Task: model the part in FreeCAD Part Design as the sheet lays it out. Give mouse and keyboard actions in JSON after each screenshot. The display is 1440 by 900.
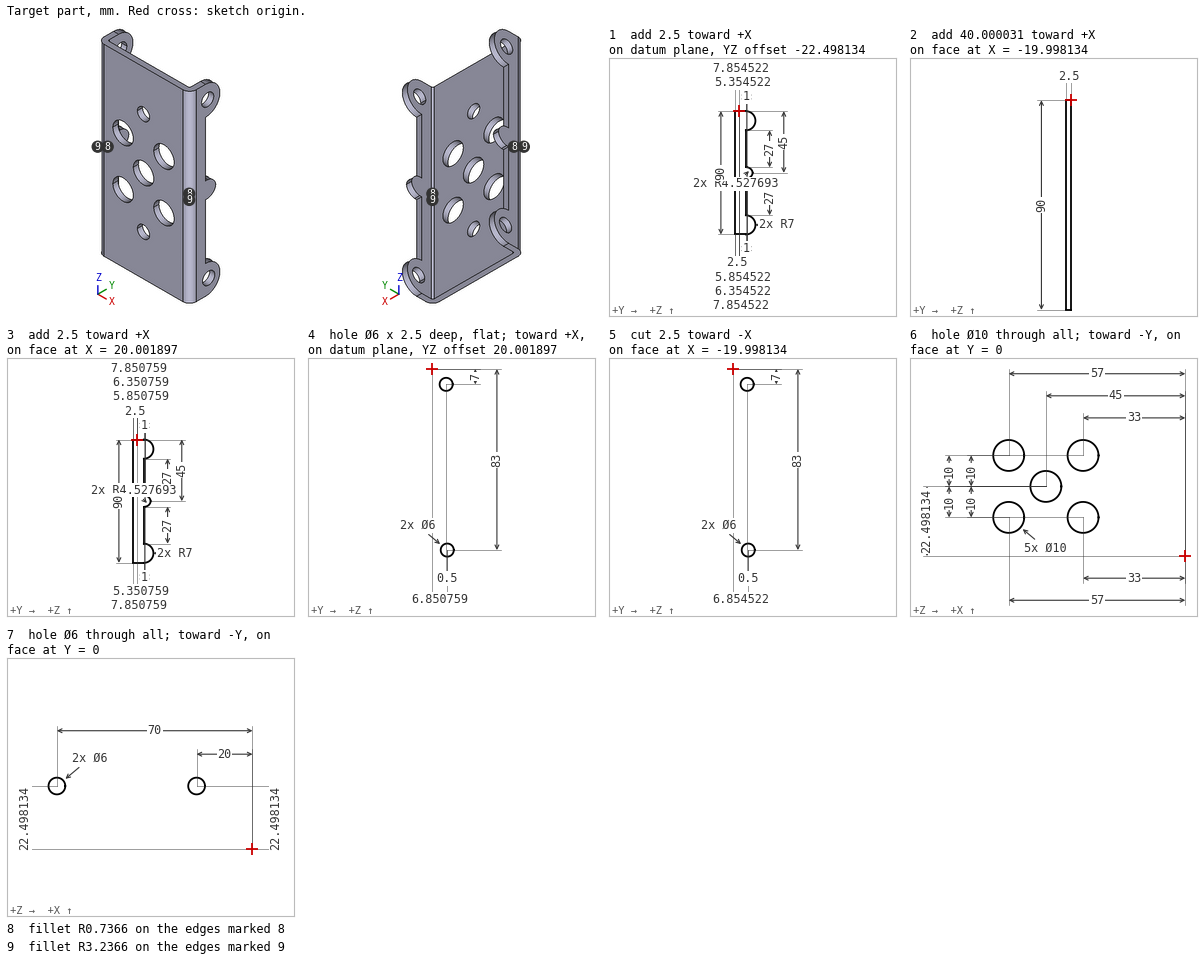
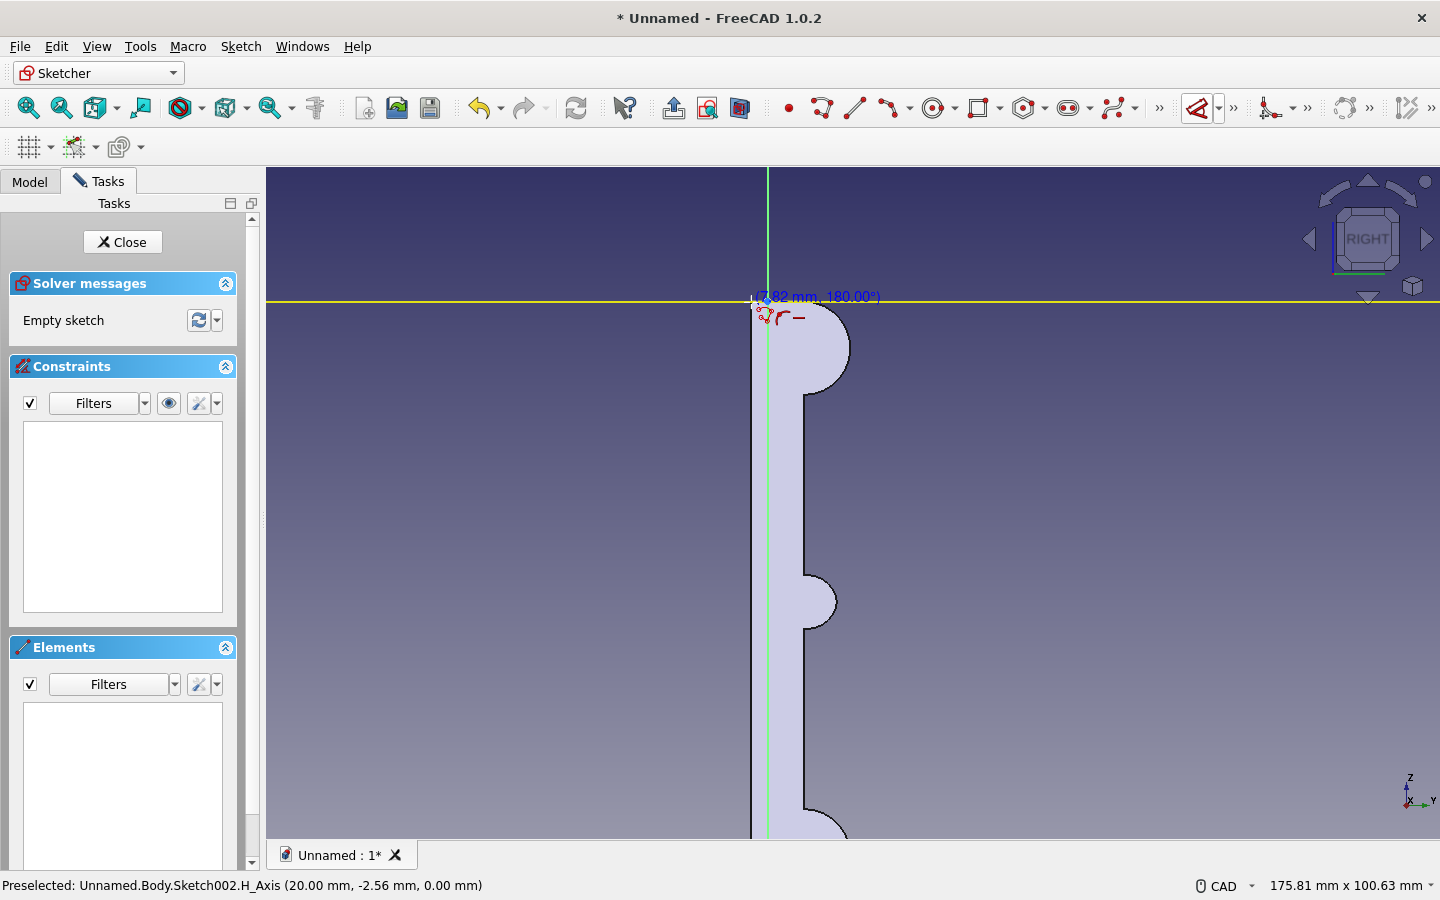
{"action": "left_click", "coordinate": [751, 311]}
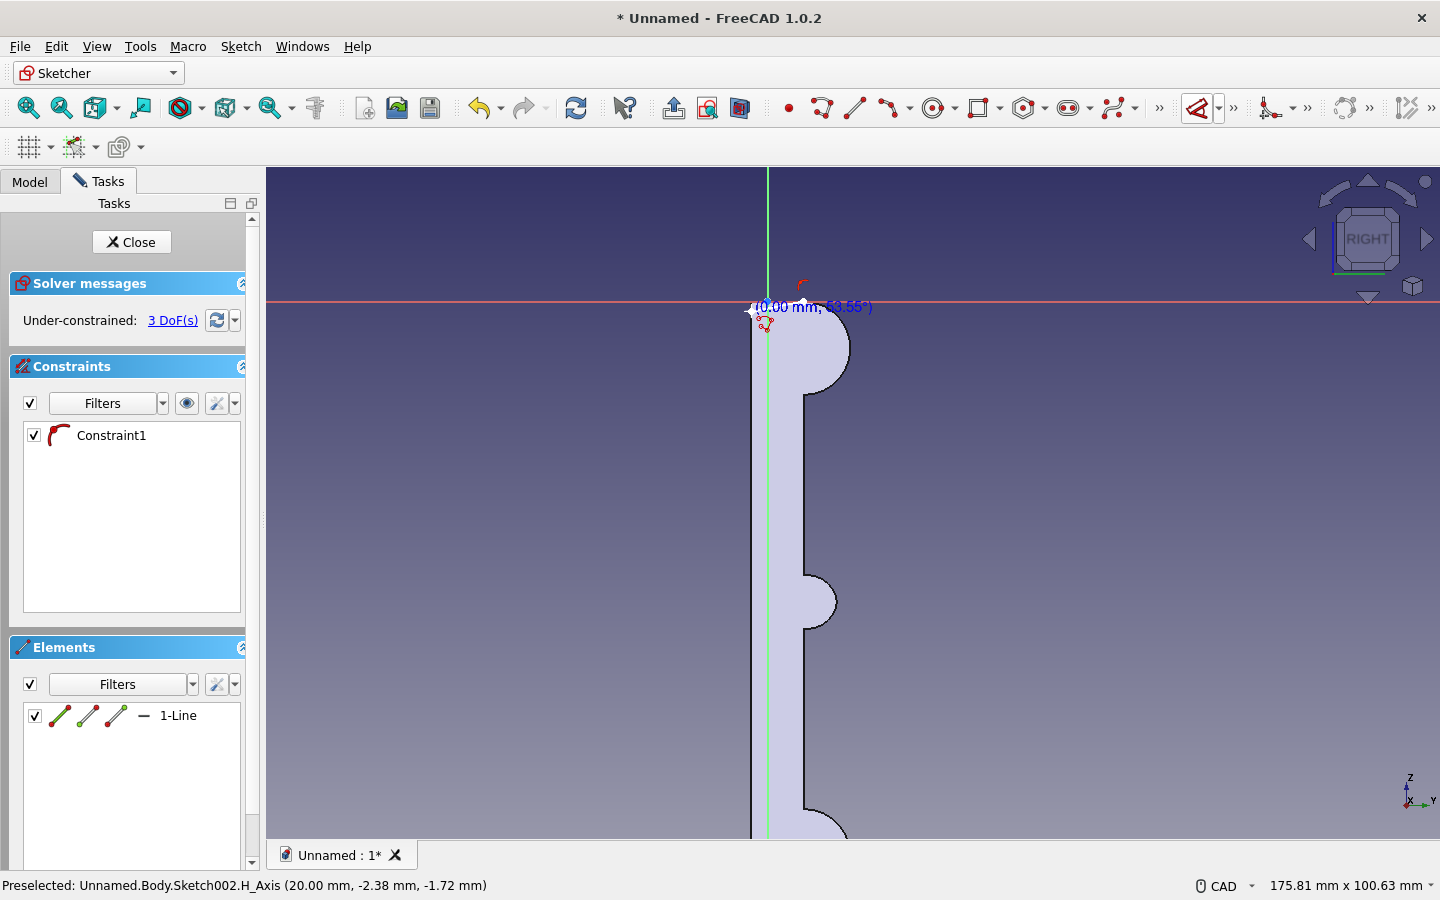
{"action": "scroll", "coordinate": [751, 302], "scroll_direction": "down", "scroll_amount": 2}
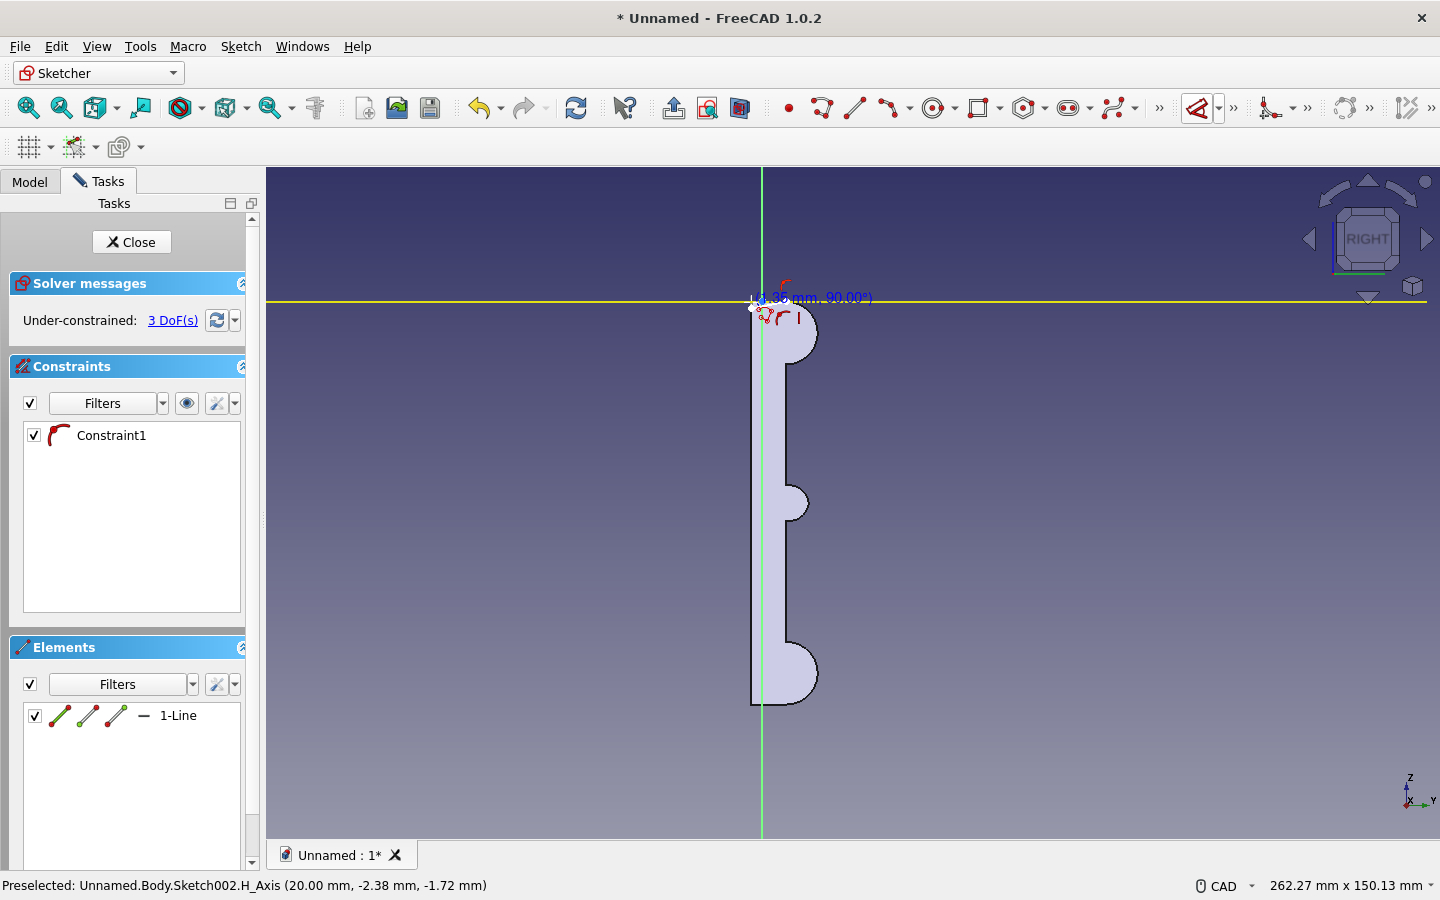
{"action": "scroll", "coordinate": [751, 705], "scroll_direction": "up", "scroll_amount": 2}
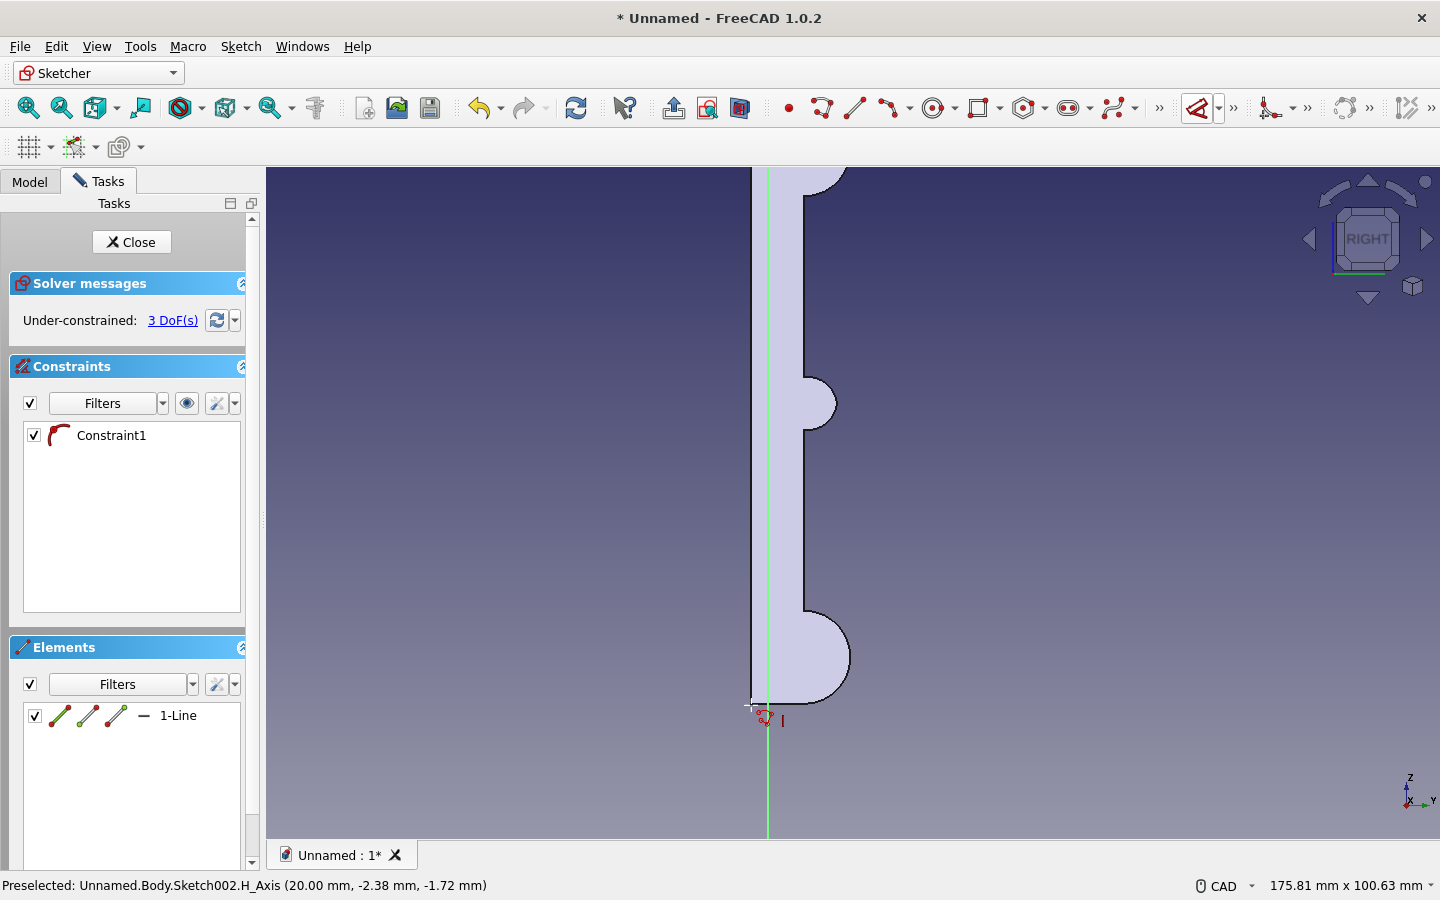
{"action": "left_click", "coordinate": [751, 704]}
{"action": "left_click", "coordinate": [804, 704]}
{"action": "right_click", "coordinate": [804, 704]}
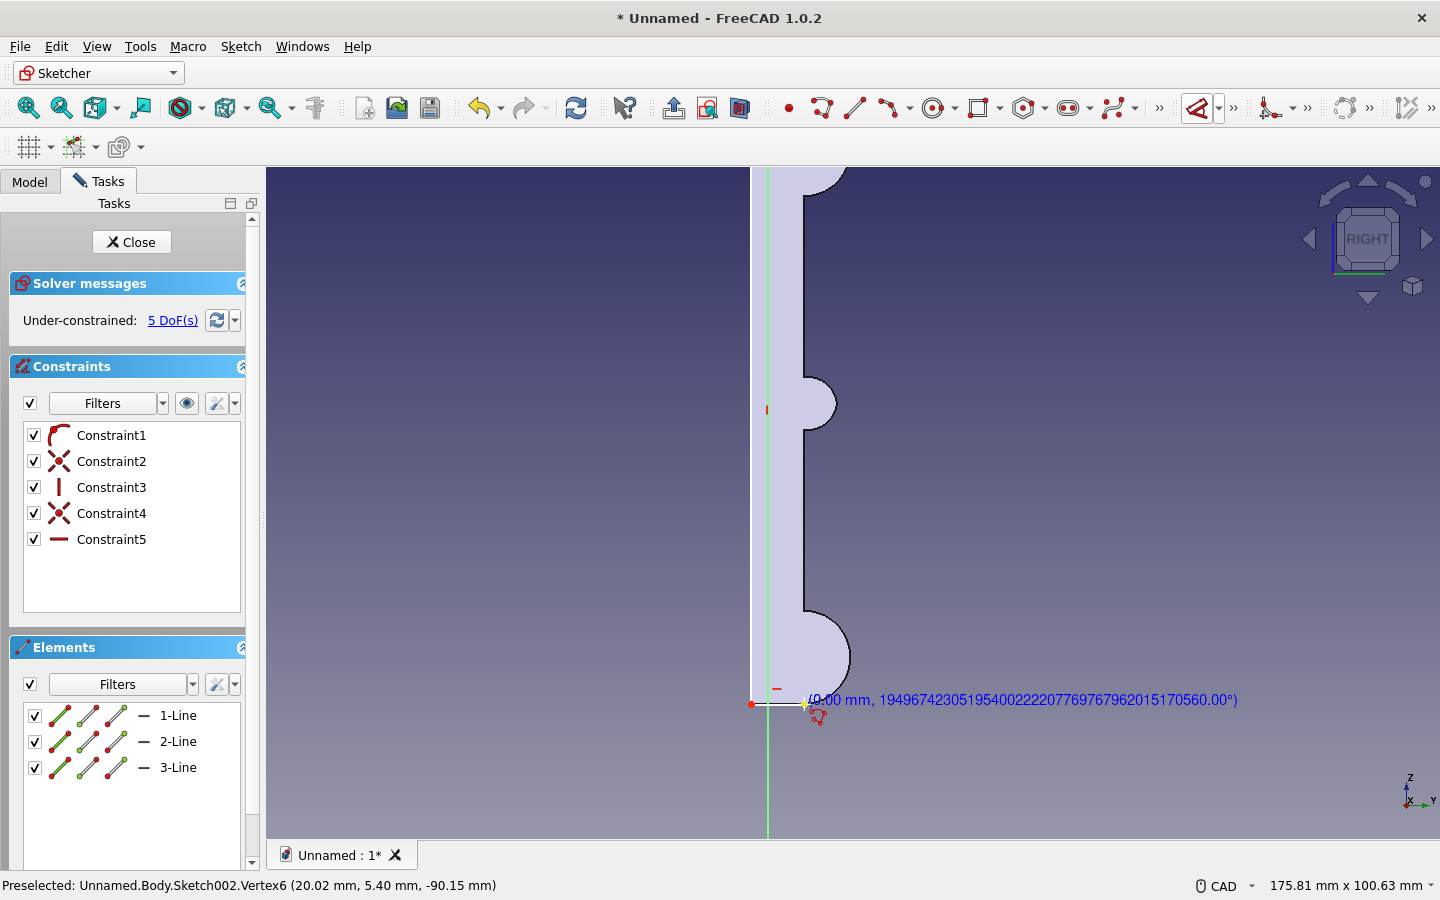
{"action": "left_click", "coordinate": [804, 611]}
{"action": "left_click", "coordinate": [804, 430]}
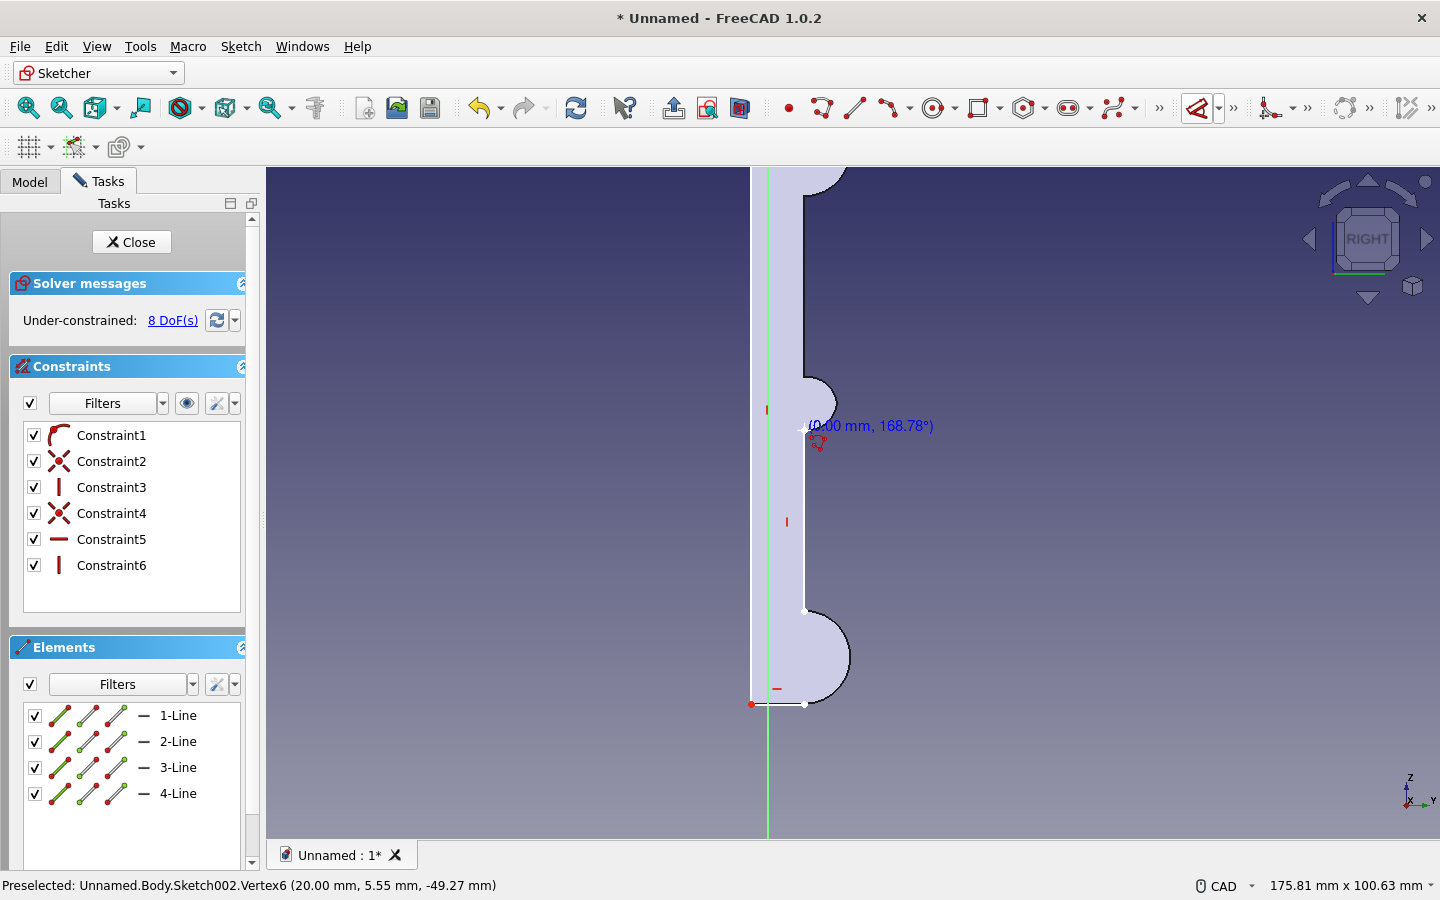
{"action": "scroll", "coordinate": [810, 430], "scroll_direction": "up", "scroll_amount": 5}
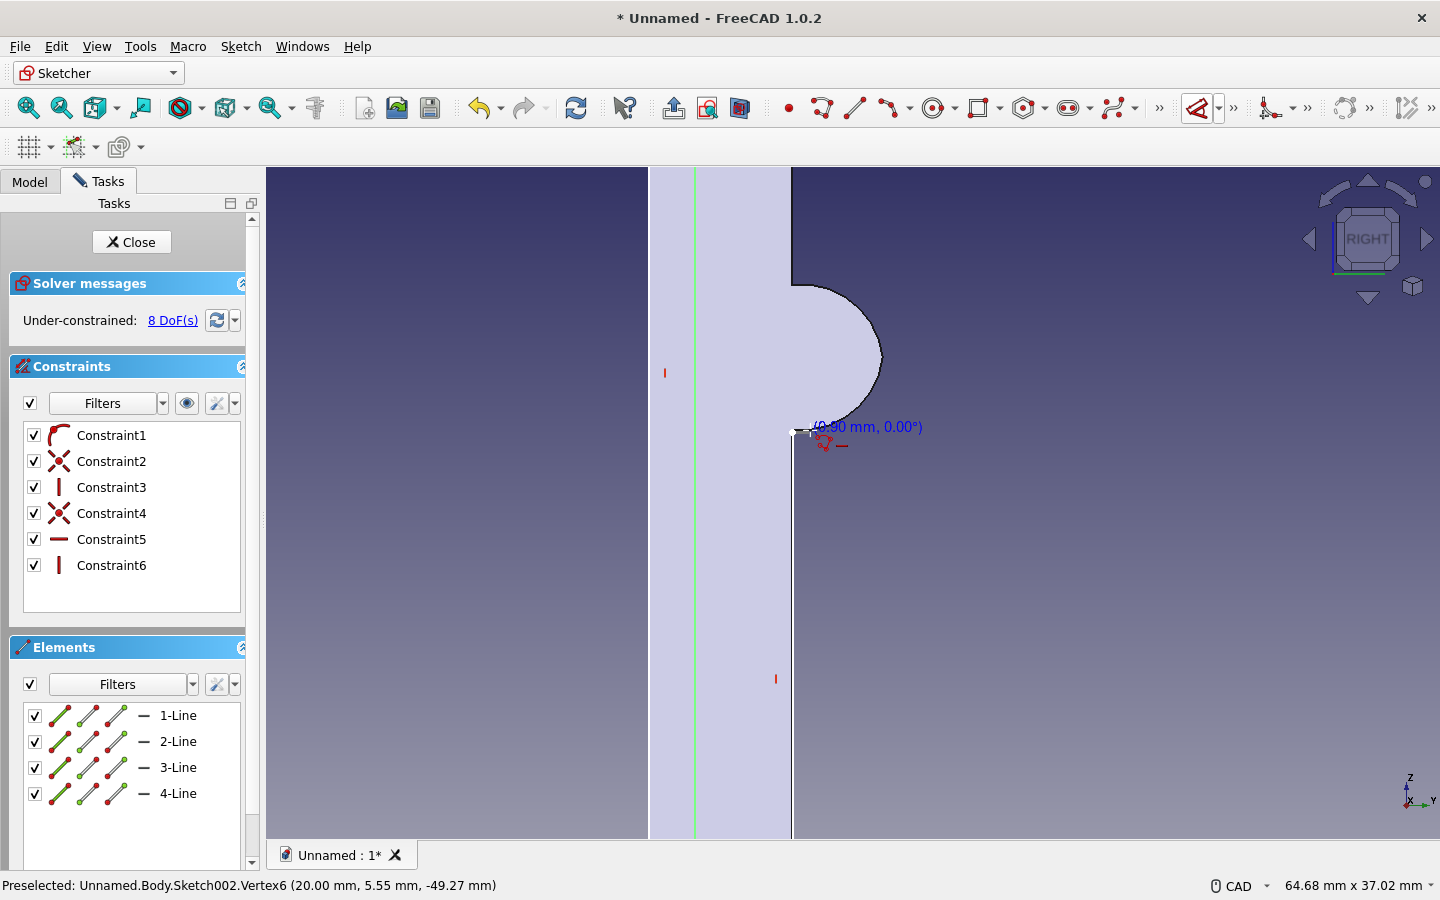
{"action": "left_click", "coordinate": [810, 429]}
{"action": "right_click", "coordinate": [810, 429]}